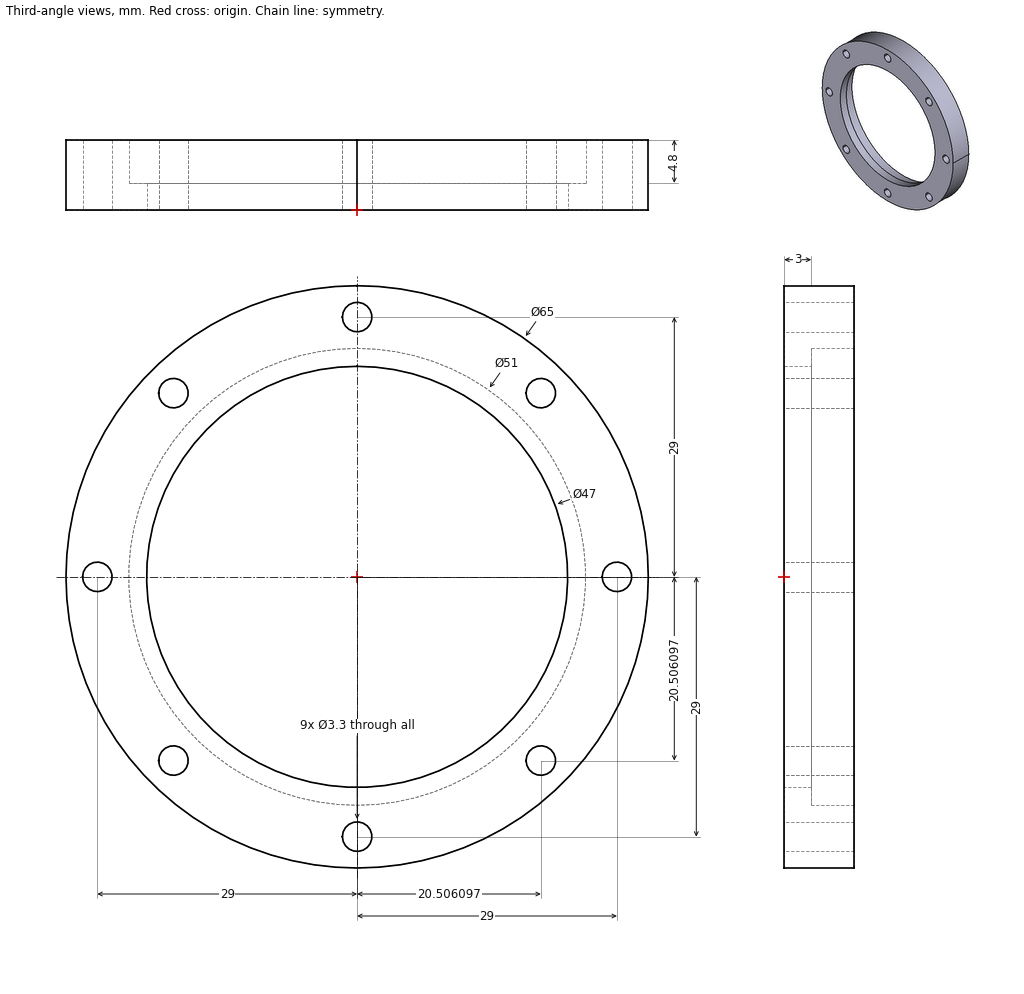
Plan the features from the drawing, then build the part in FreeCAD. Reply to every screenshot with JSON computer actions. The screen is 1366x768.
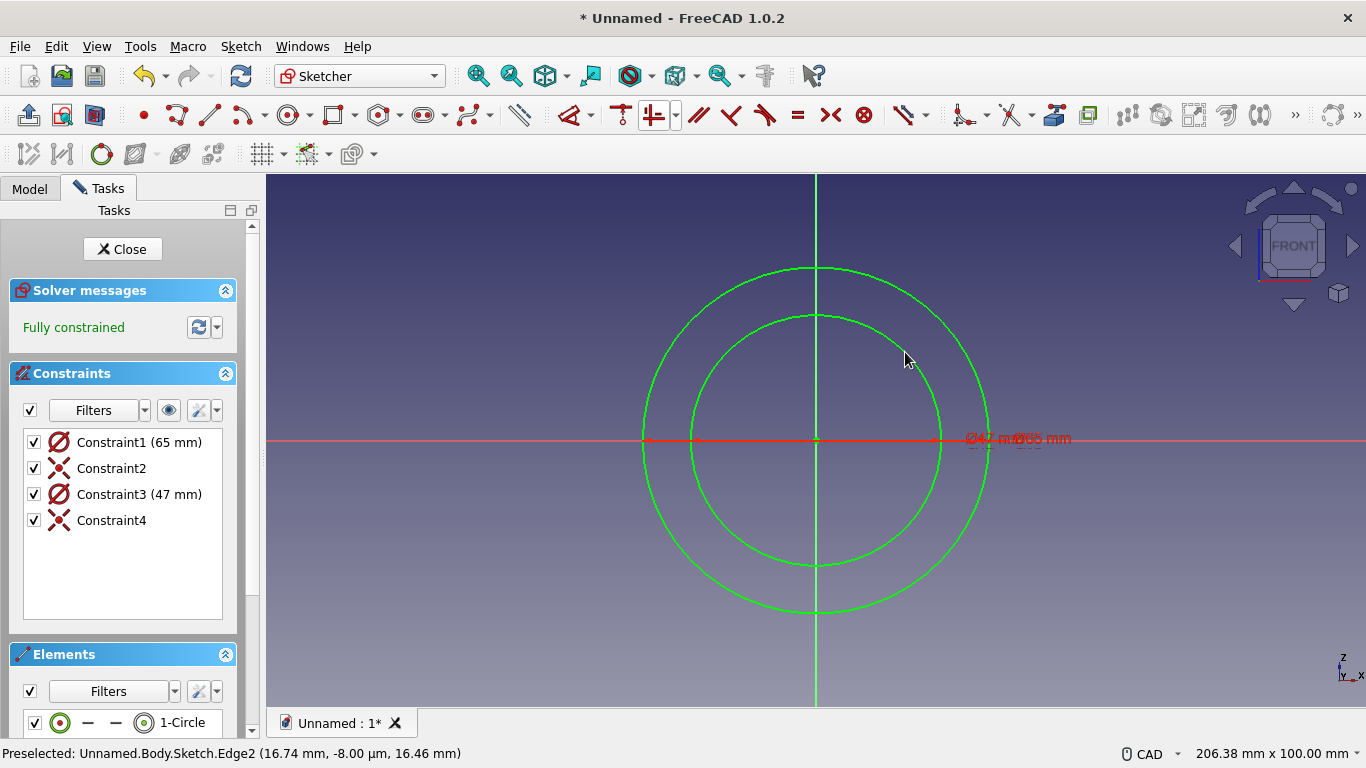
{"action": "left_click", "coordinate": [123, 249]}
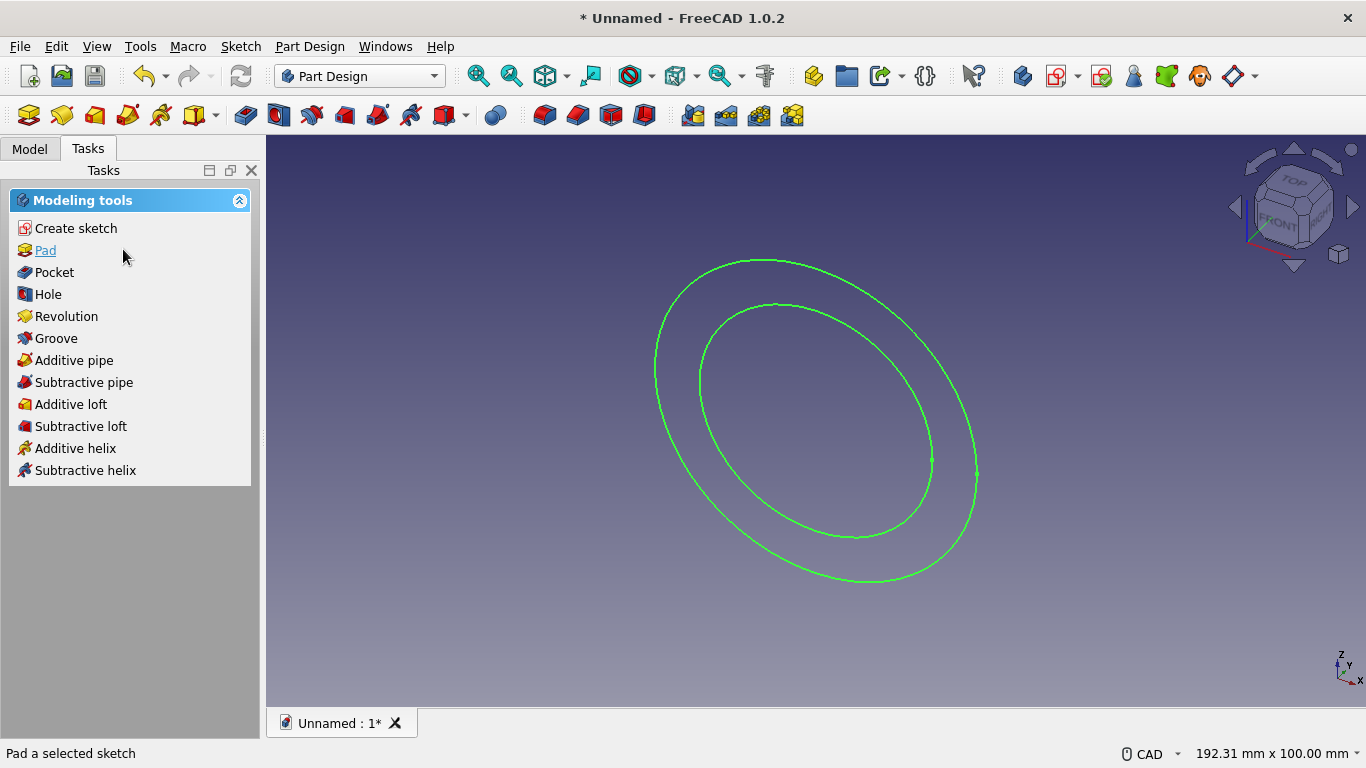
{"action": "left_click", "coordinate": [29, 116]}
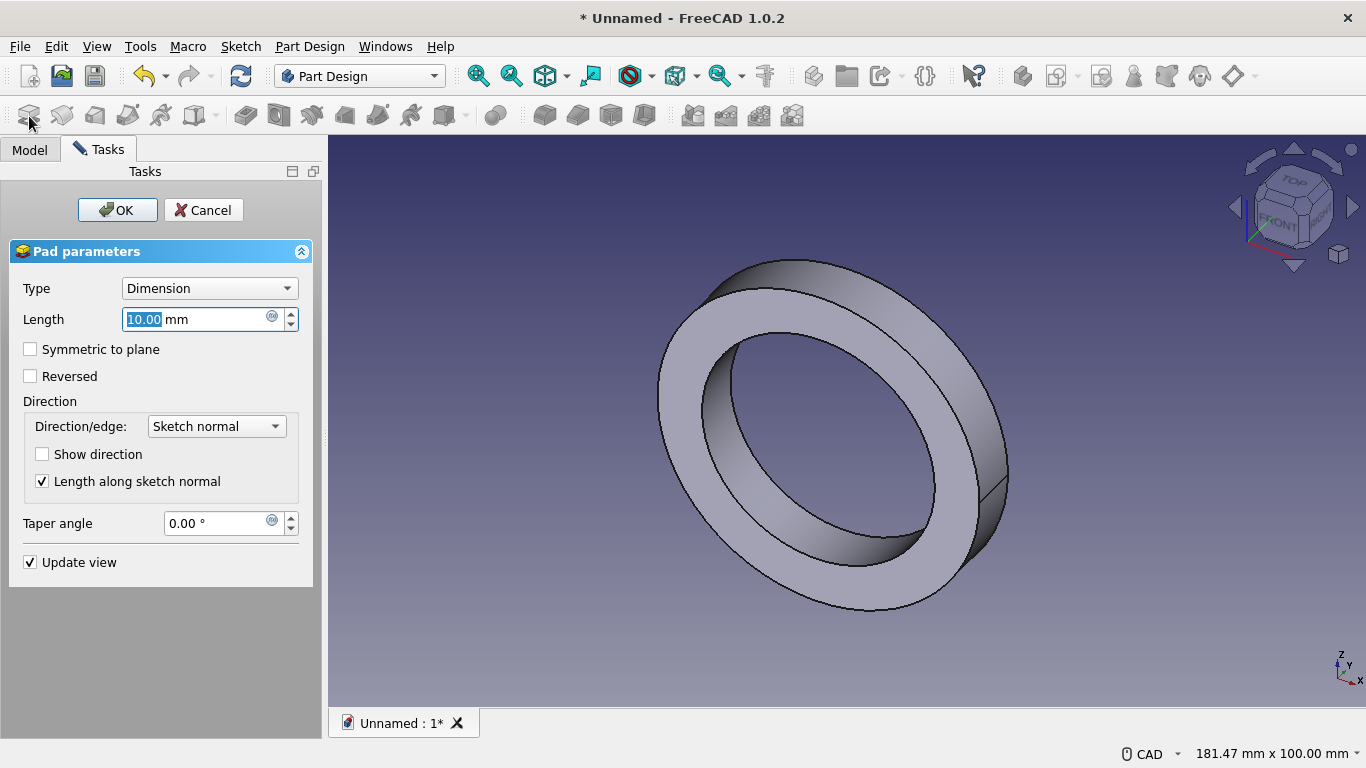
{"action": "type", "text": "3"}
{"action": "key", "text": "Tab"}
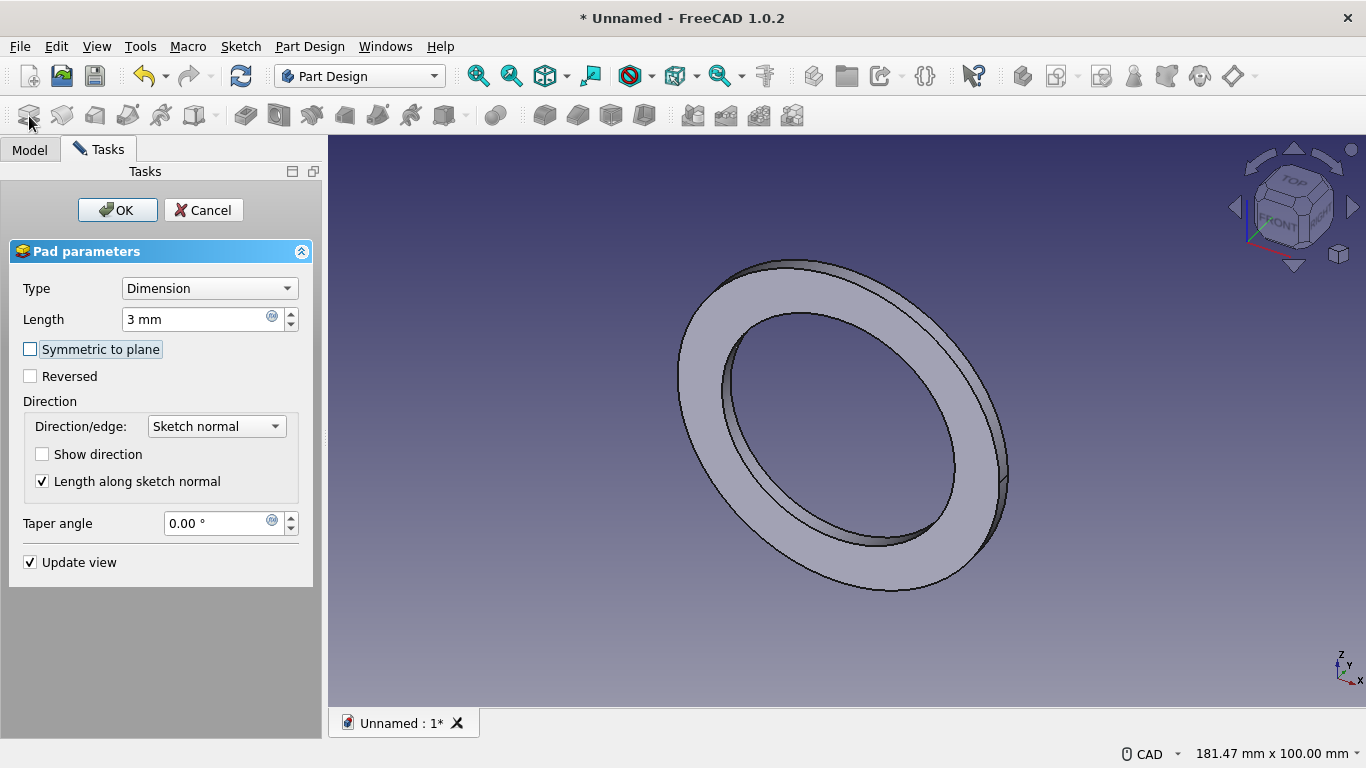
{"action": "left_click", "coordinate": [31, 376]}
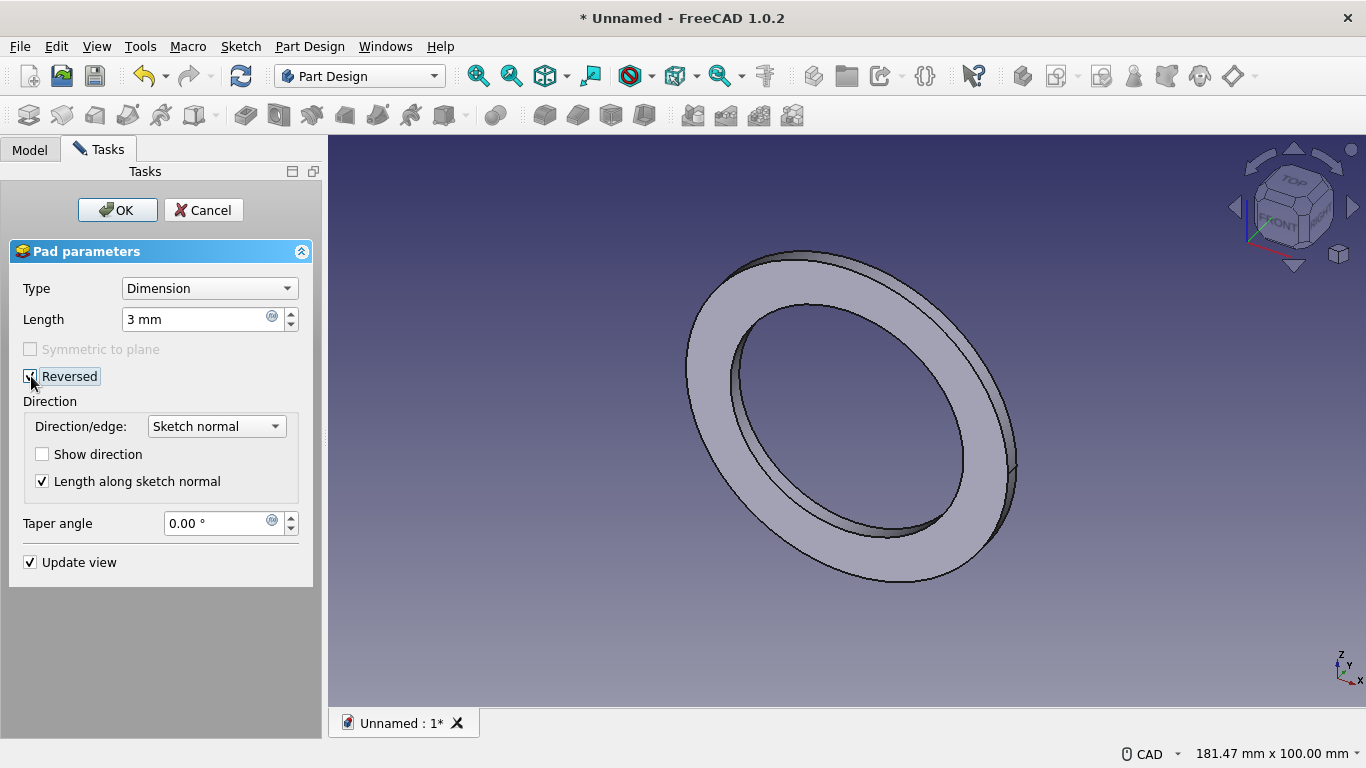
{"action": "left_click", "coordinate": [118, 210]}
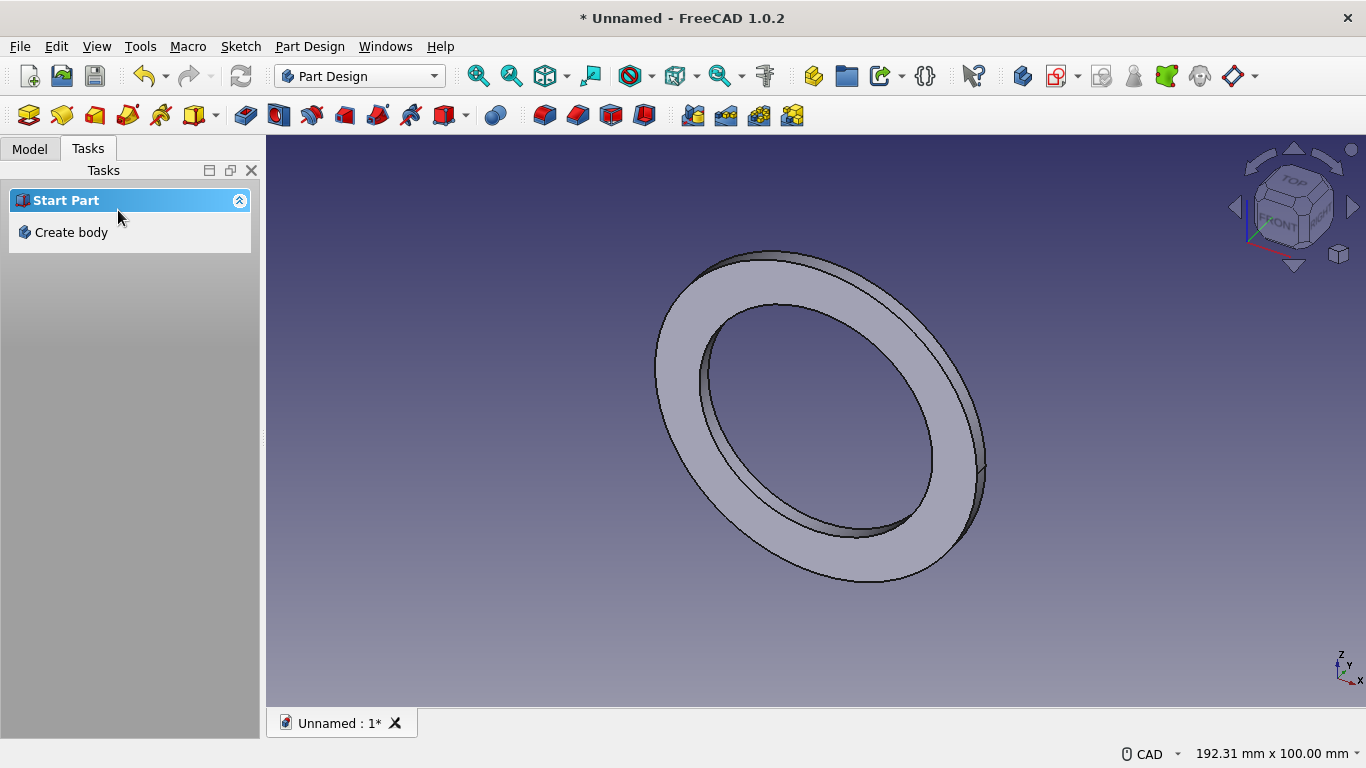
{"action": "key", "text": "4"}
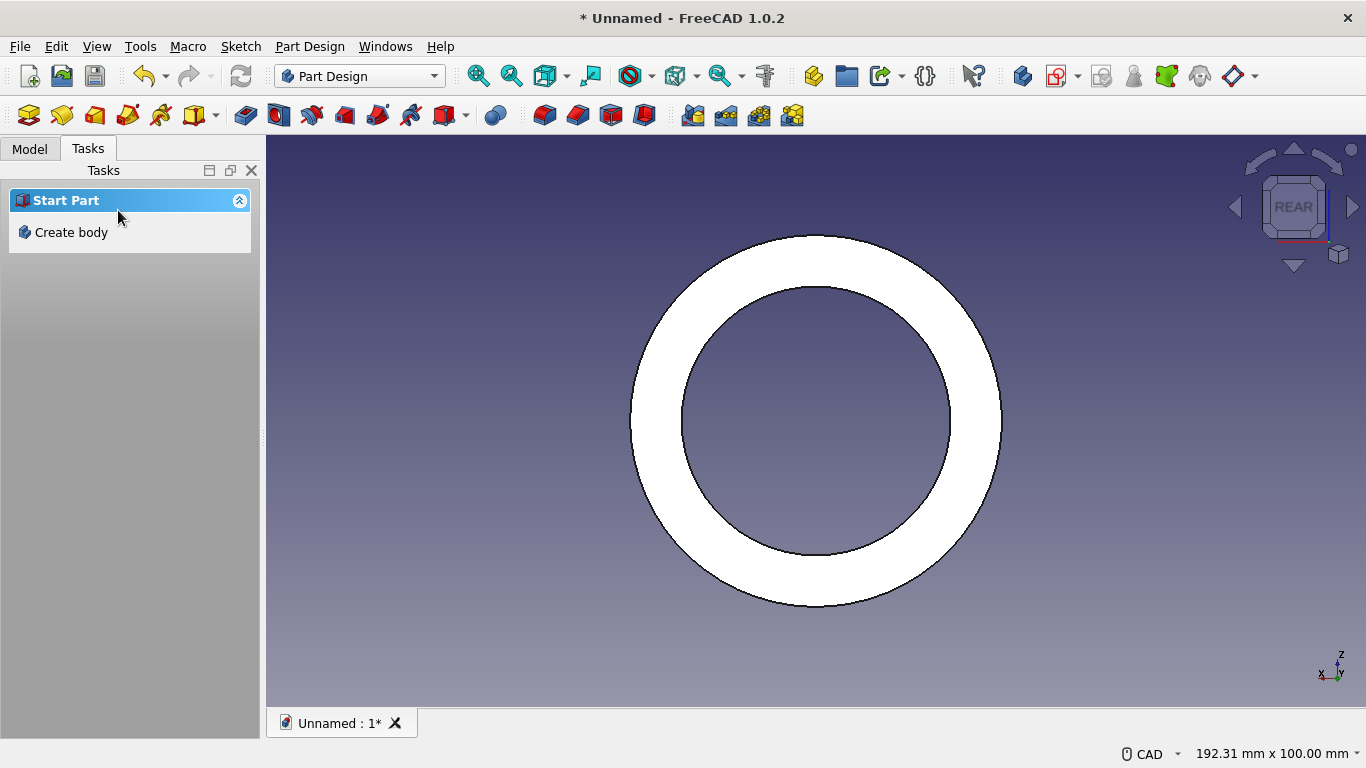
{"action": "left_click", "coordinate": [816, 579]}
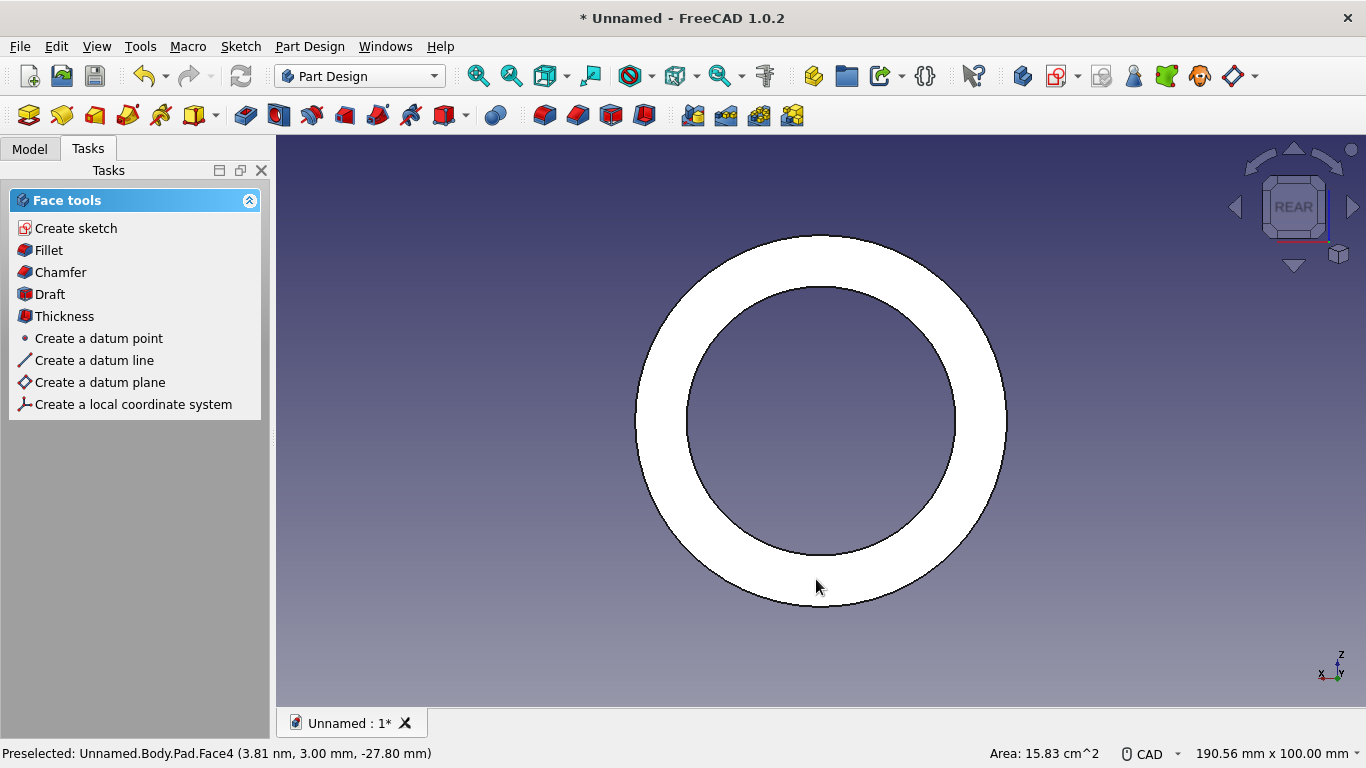
{"action": "left_click", "coordinate": [1056, 76]}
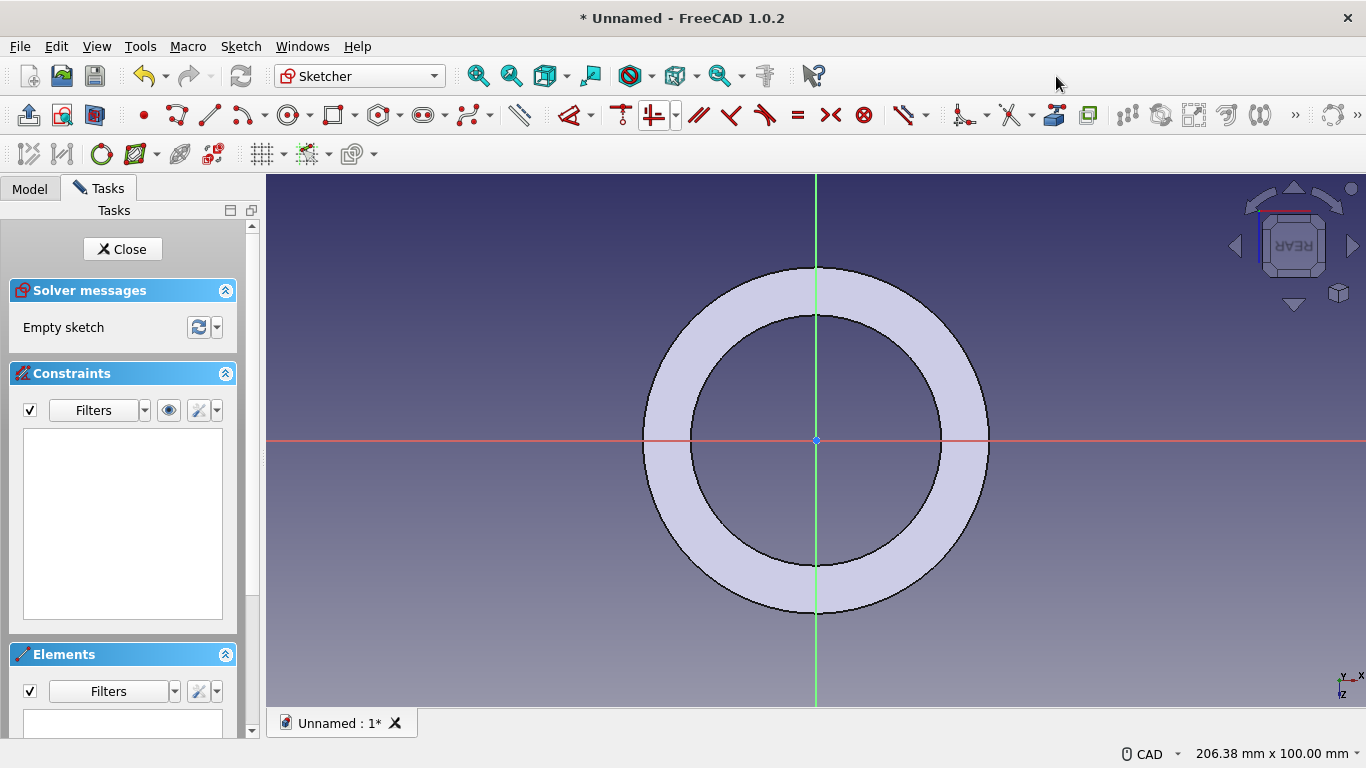
{"action": "left_click", "coordinate": [288, 116]}